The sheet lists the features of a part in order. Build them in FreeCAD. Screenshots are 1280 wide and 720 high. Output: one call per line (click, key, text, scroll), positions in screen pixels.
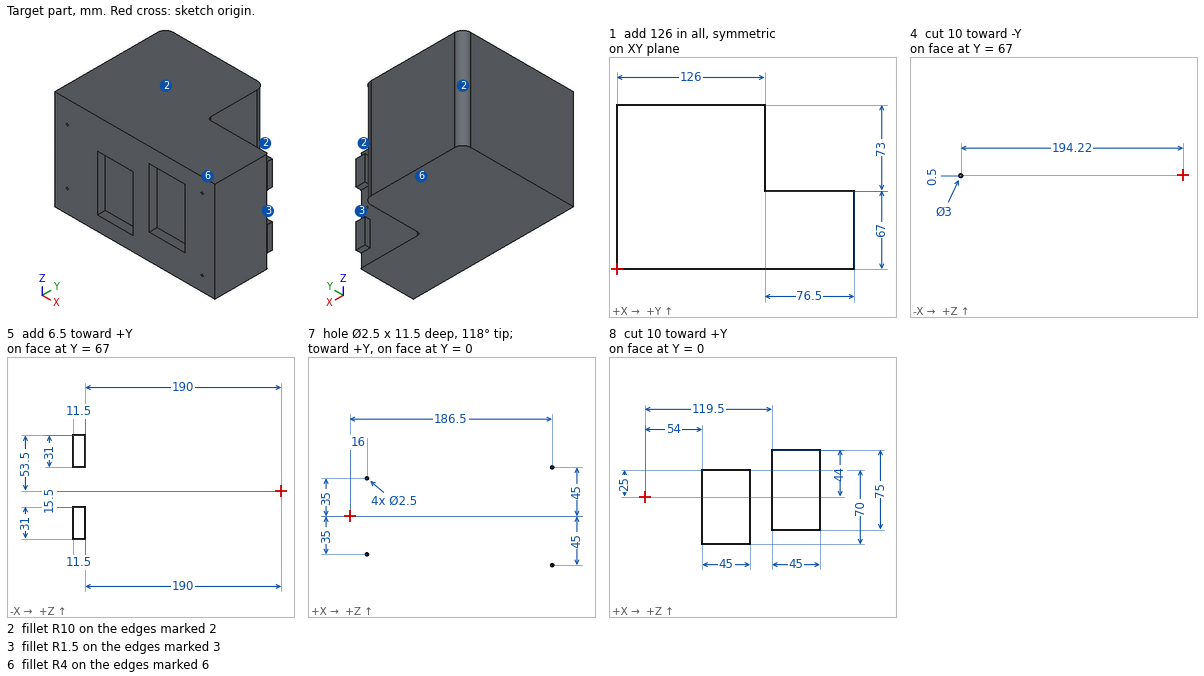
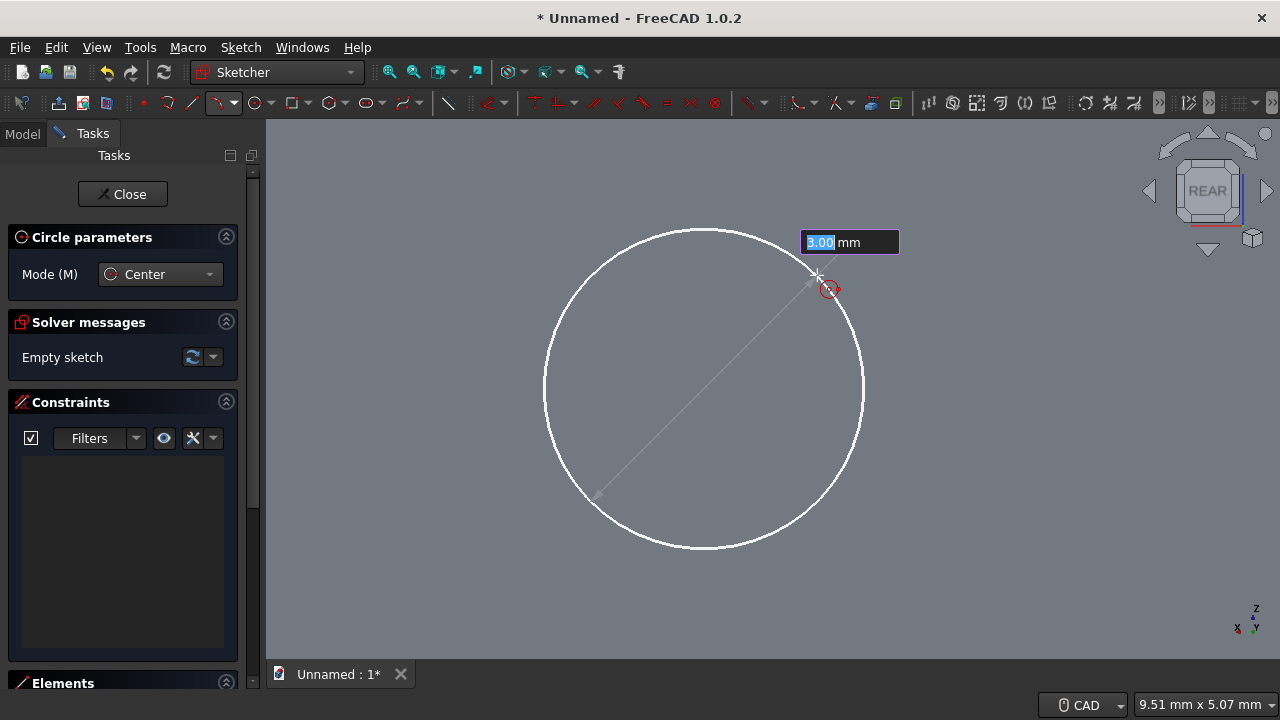
text(3)
key(Return)
key(Escape)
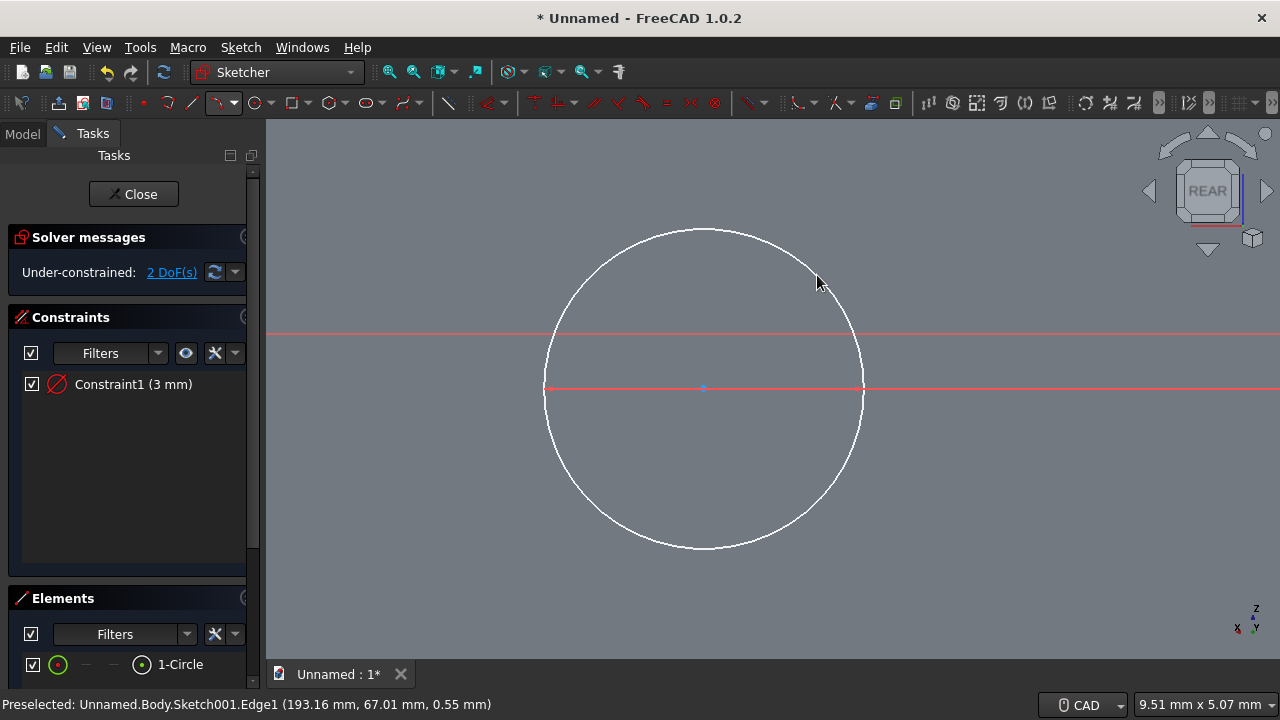
key(d)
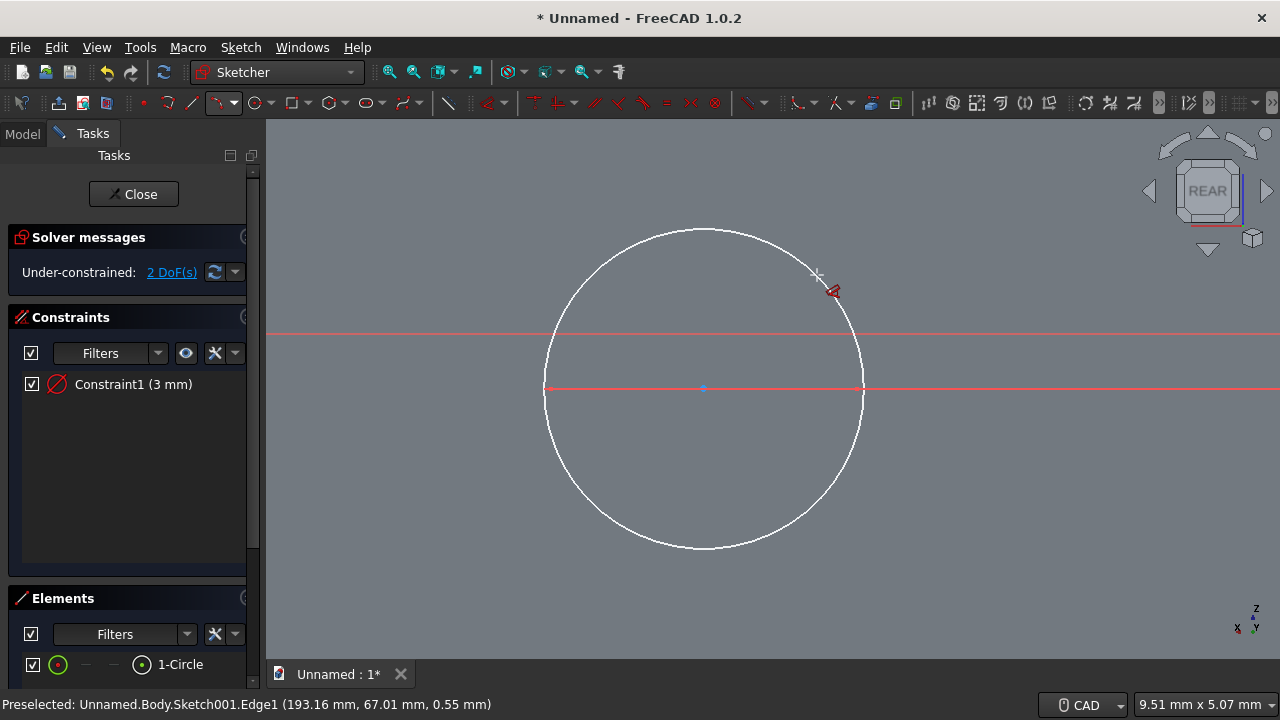
click(704, 389)
click(670, 362)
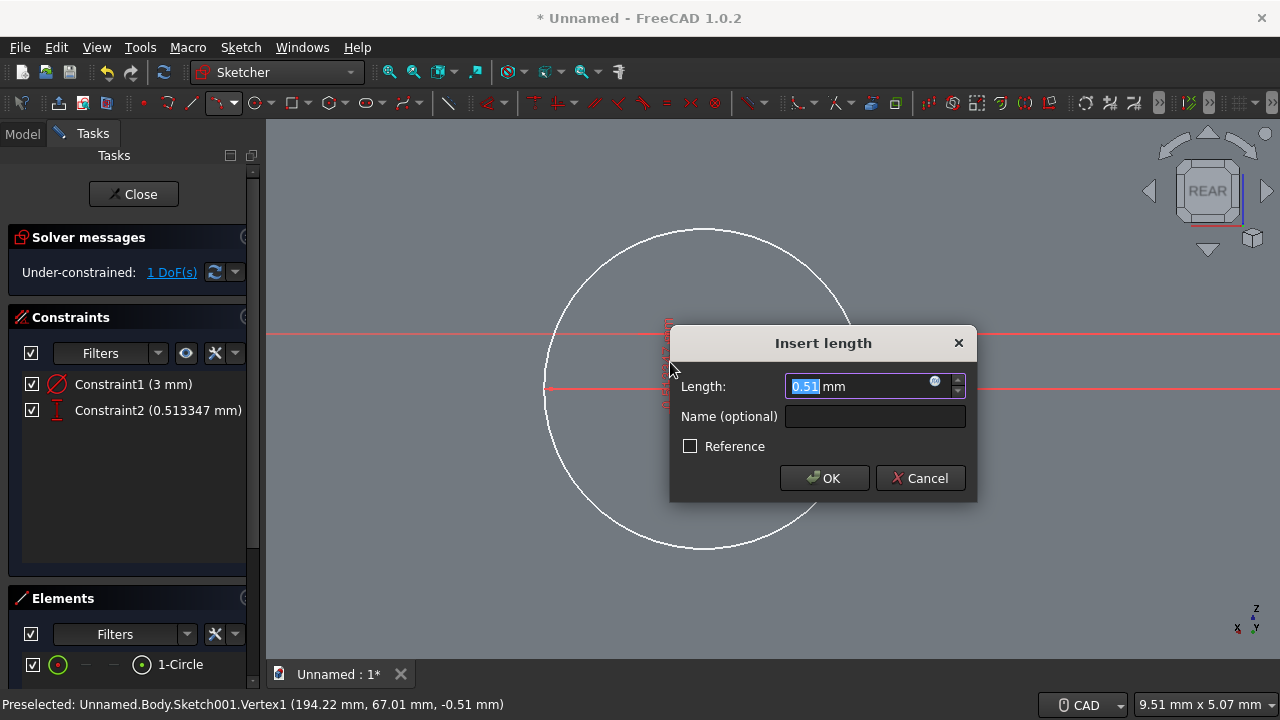
text(0.5)
key(Return)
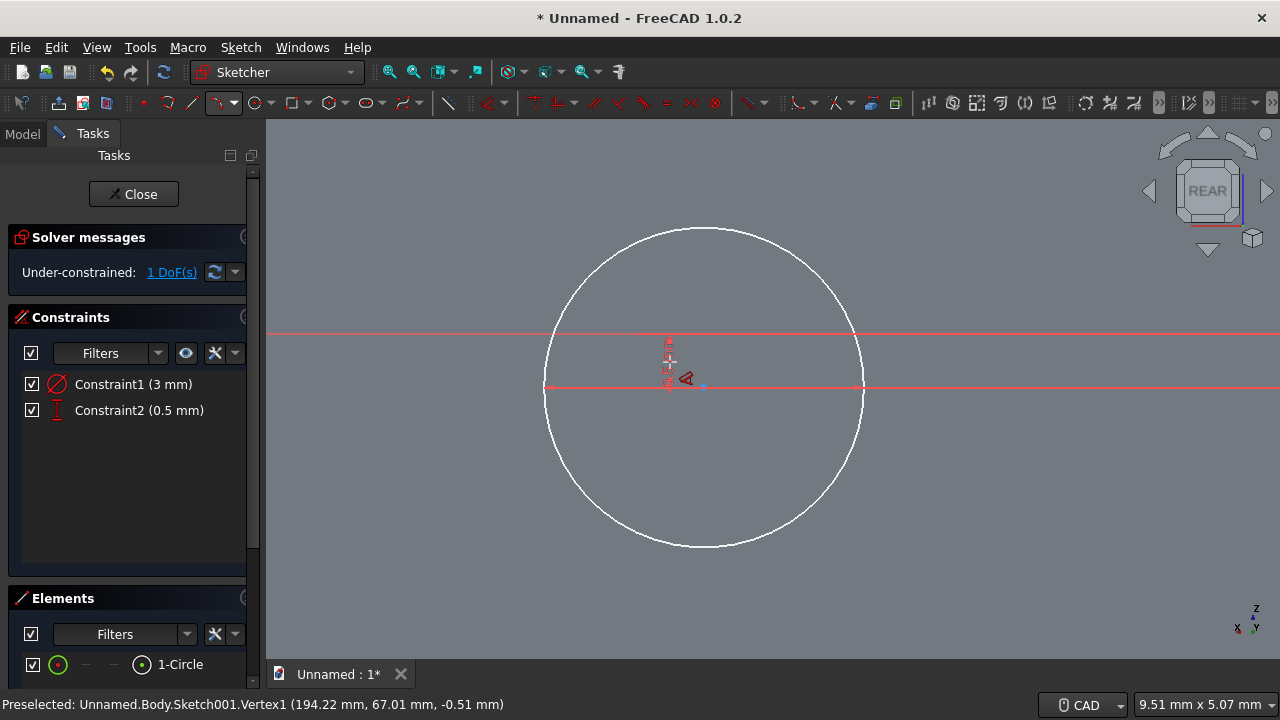
click(704, 388)
click(909, 300)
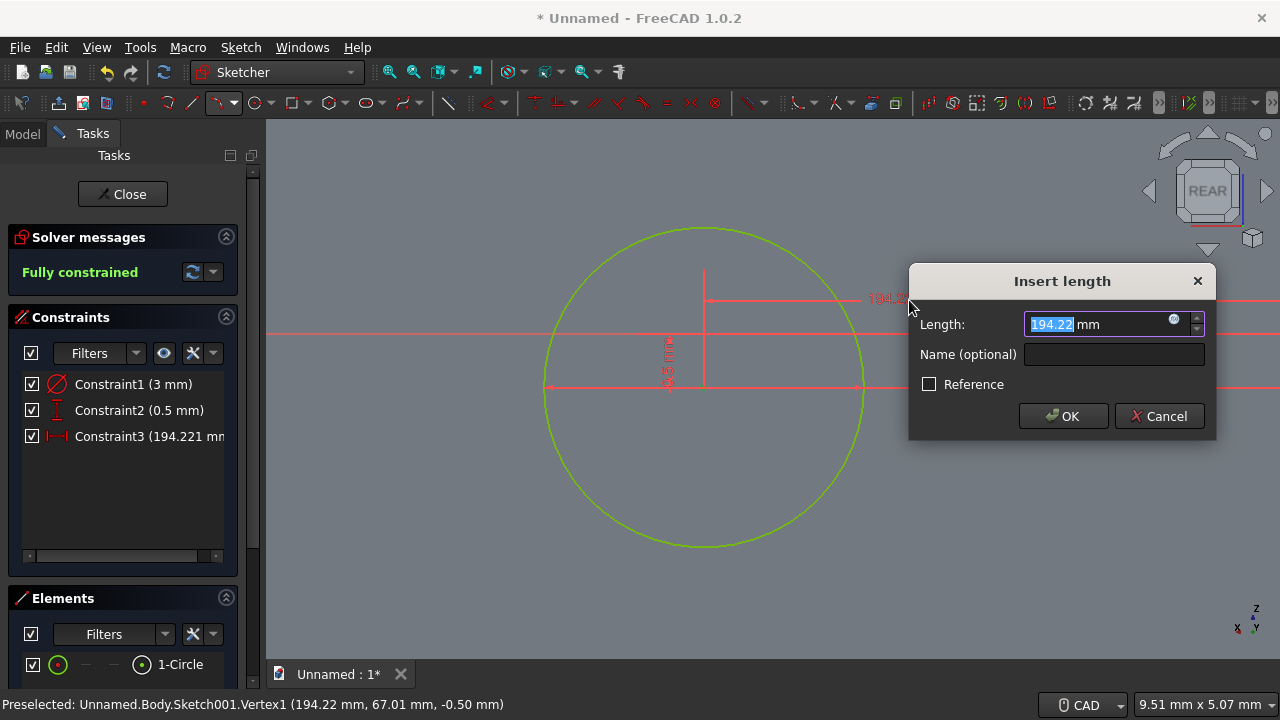
text(194.22)
key(Return)
key(Escape)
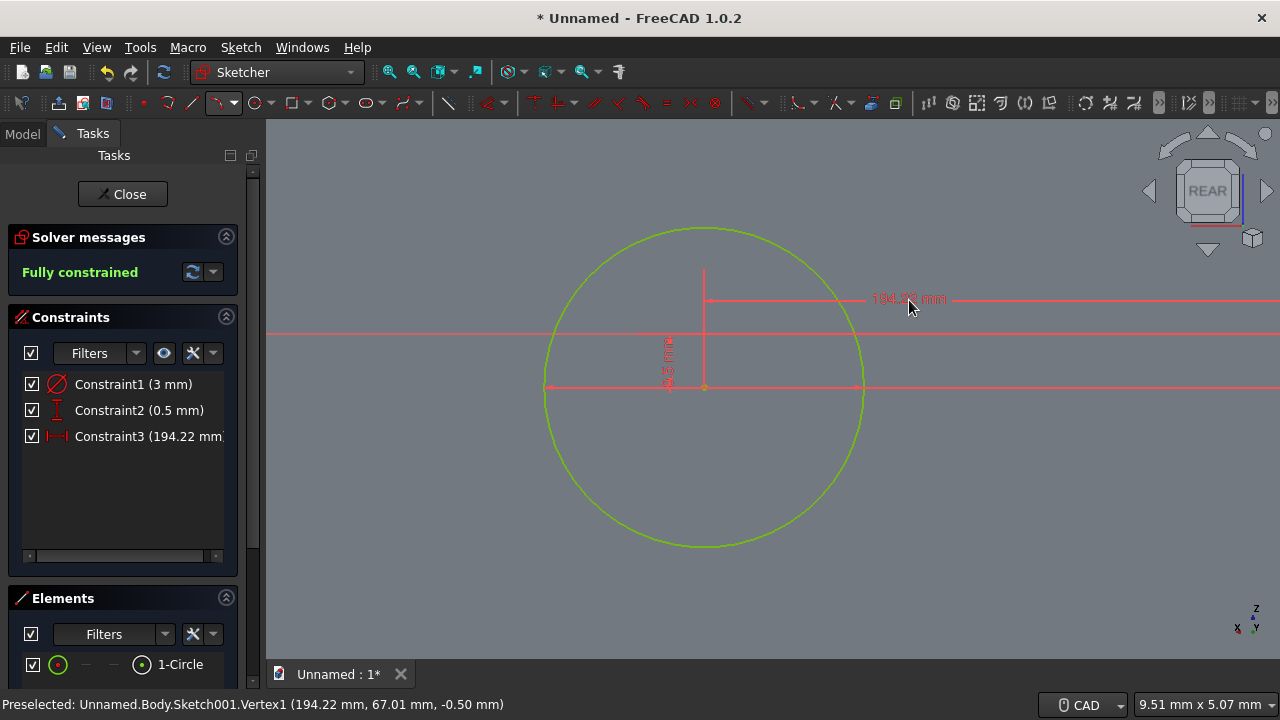
click(123, 194)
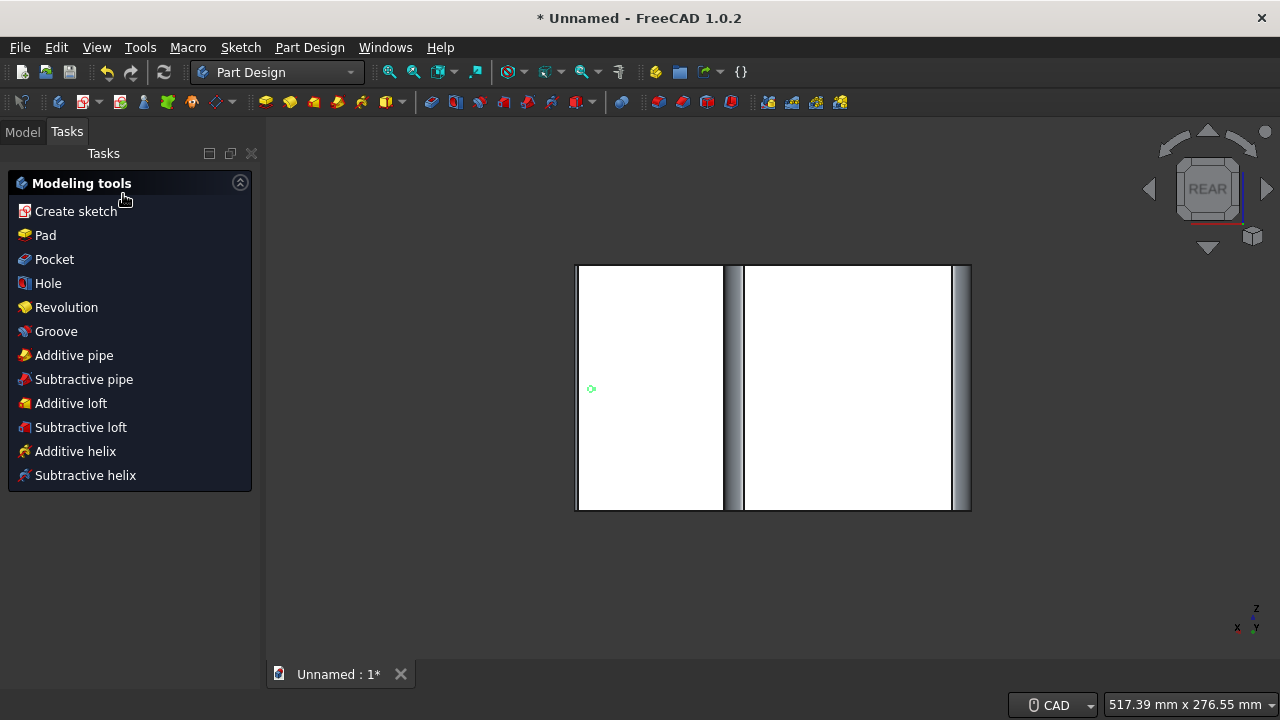
click(432, 102)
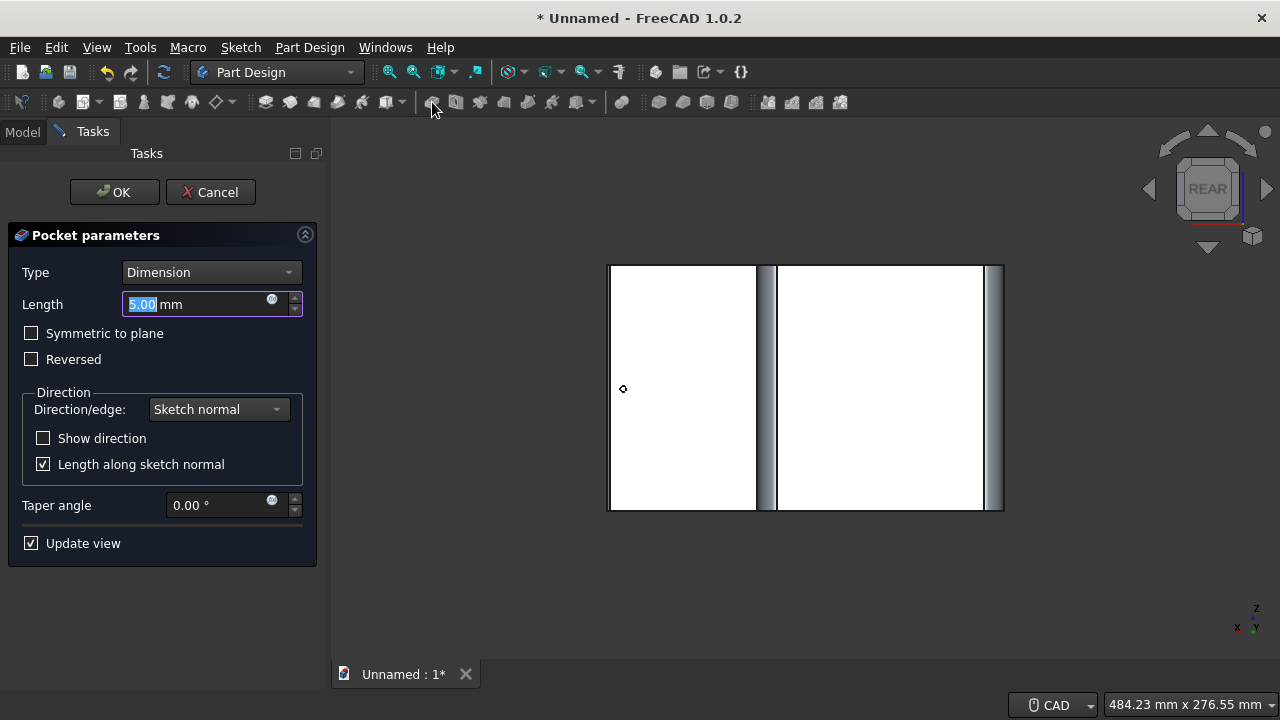
text(10)
key(Tab)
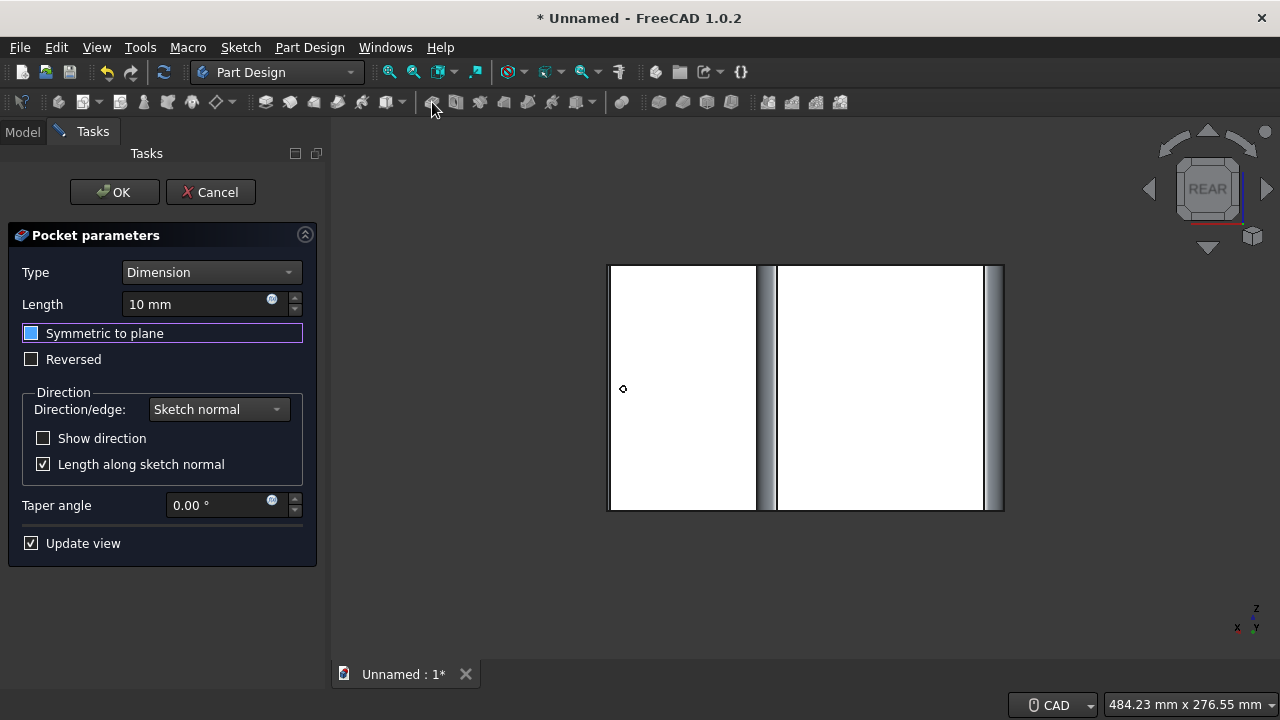
click(115, 192)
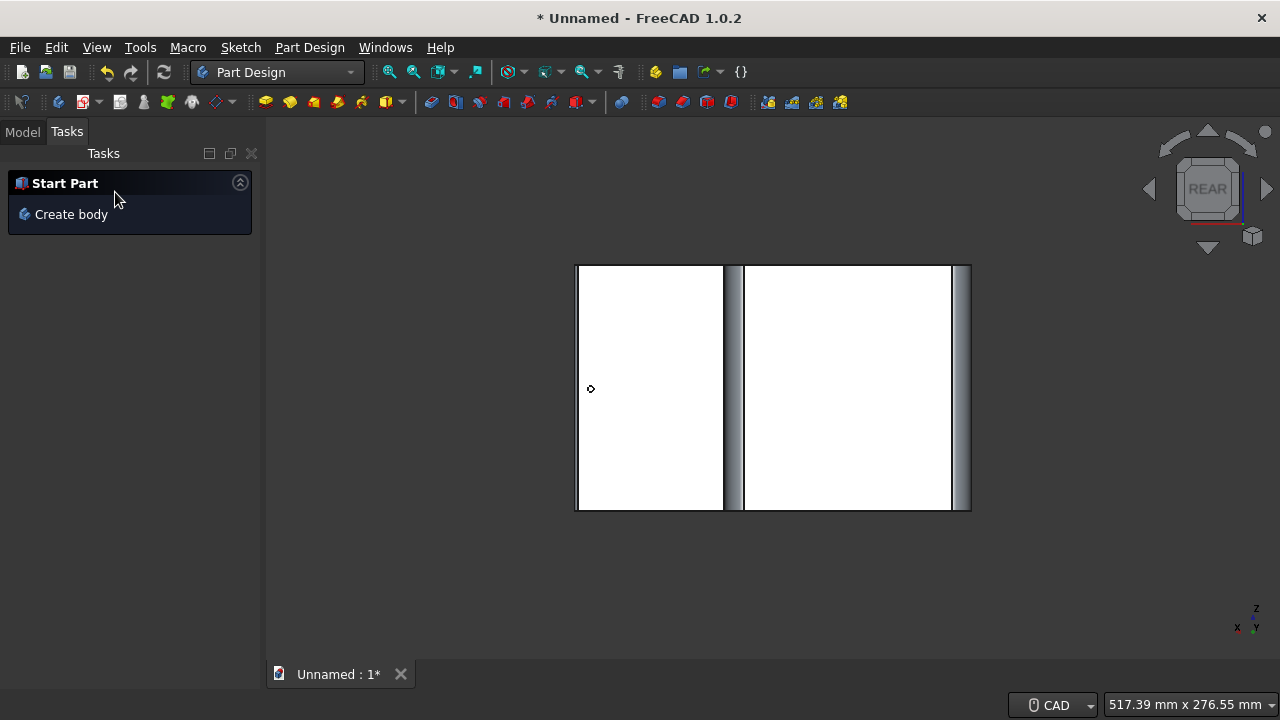
click(651, 352)